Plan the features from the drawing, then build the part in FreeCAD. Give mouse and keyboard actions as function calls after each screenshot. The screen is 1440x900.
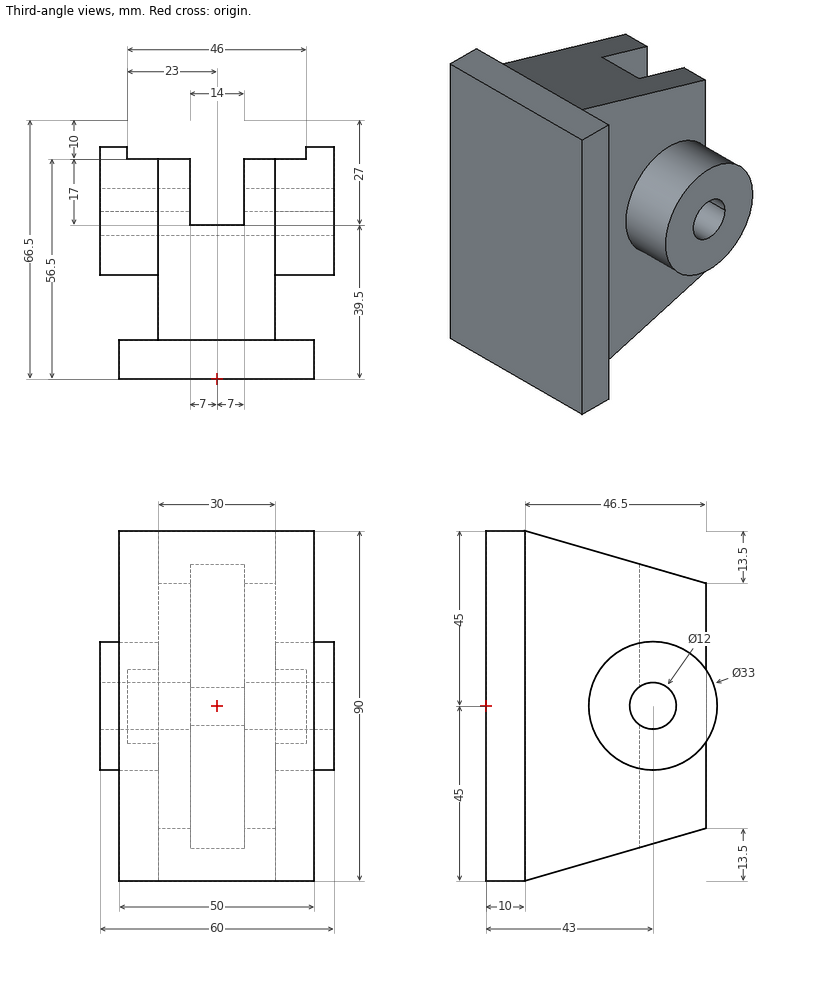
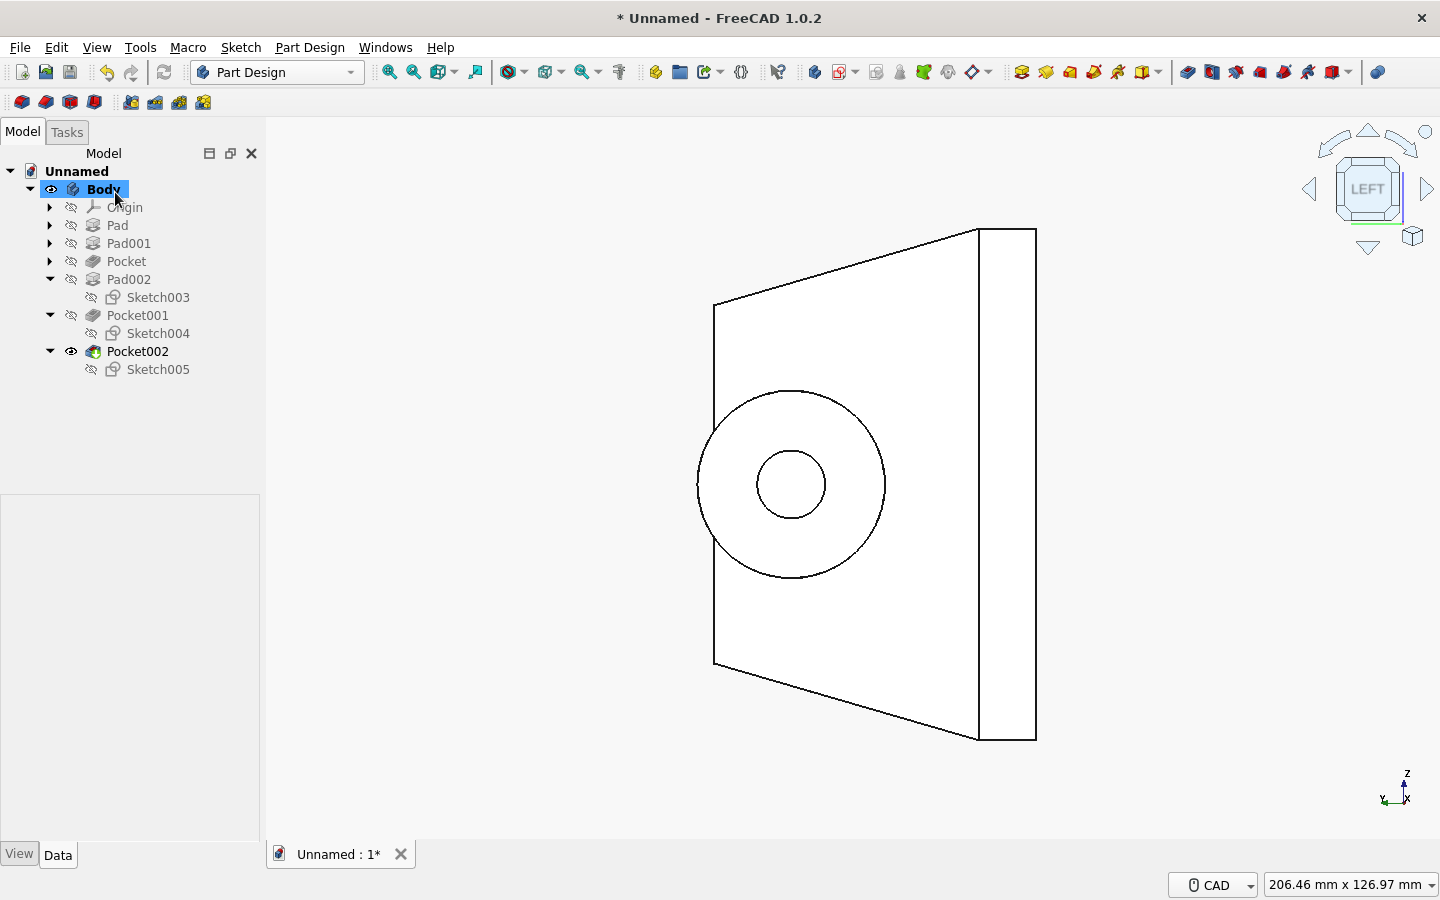
click(884, 630)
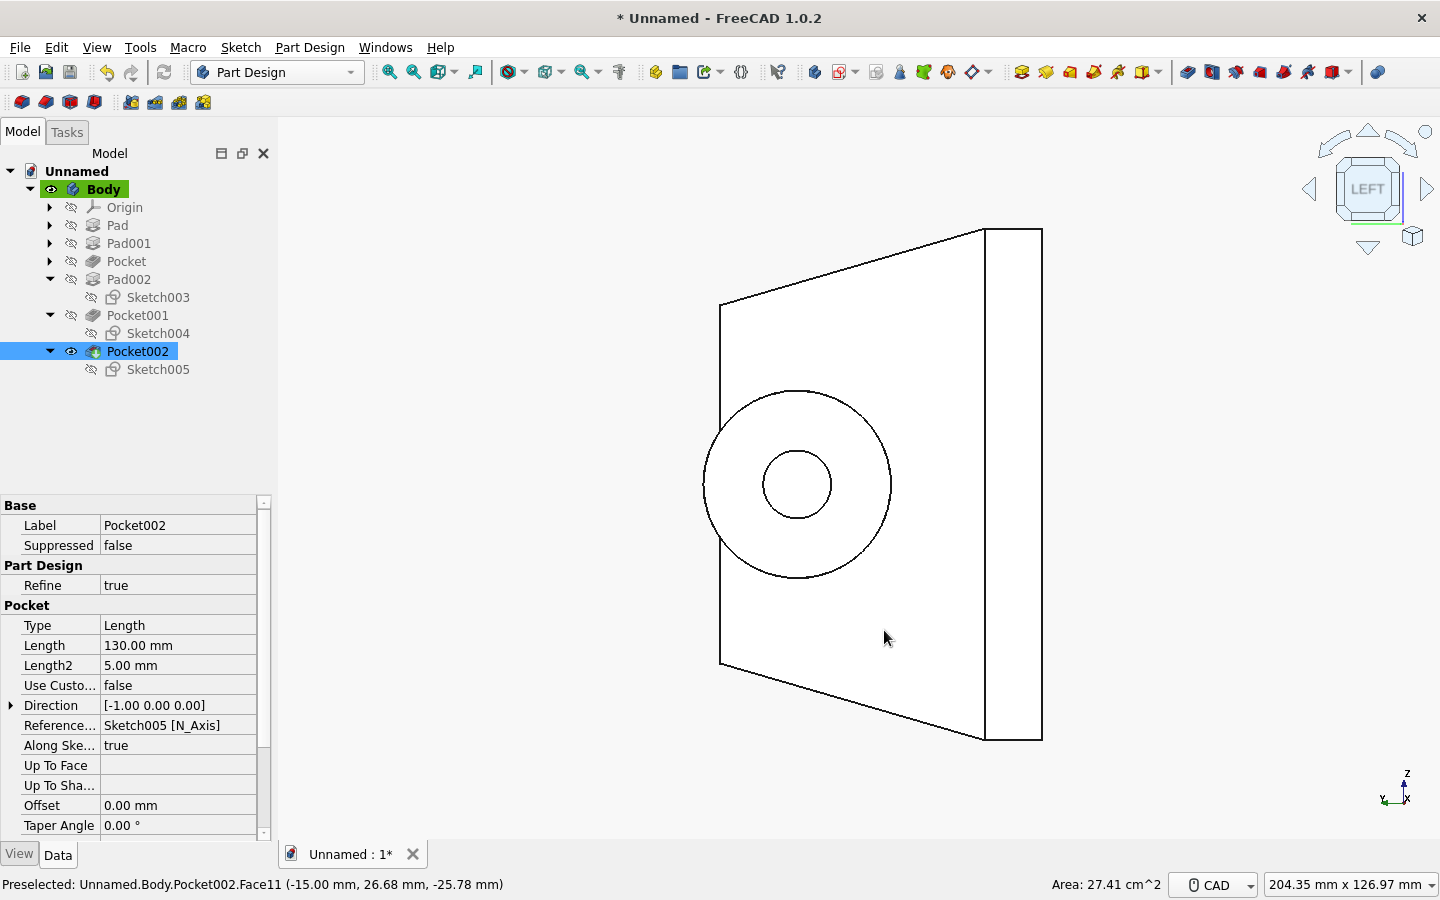
click(840, 72)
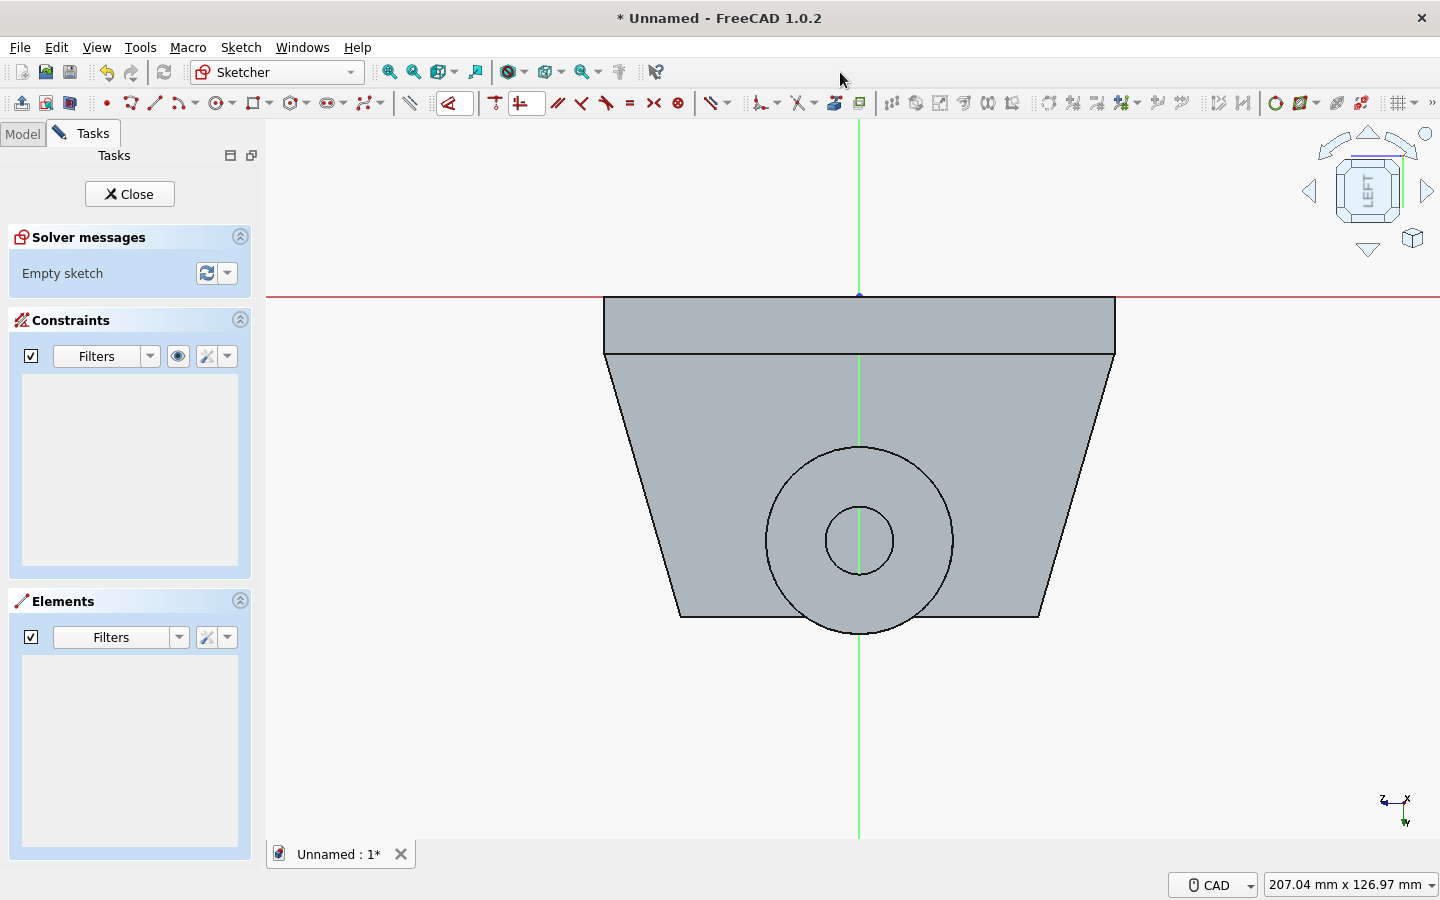
click(70, 104)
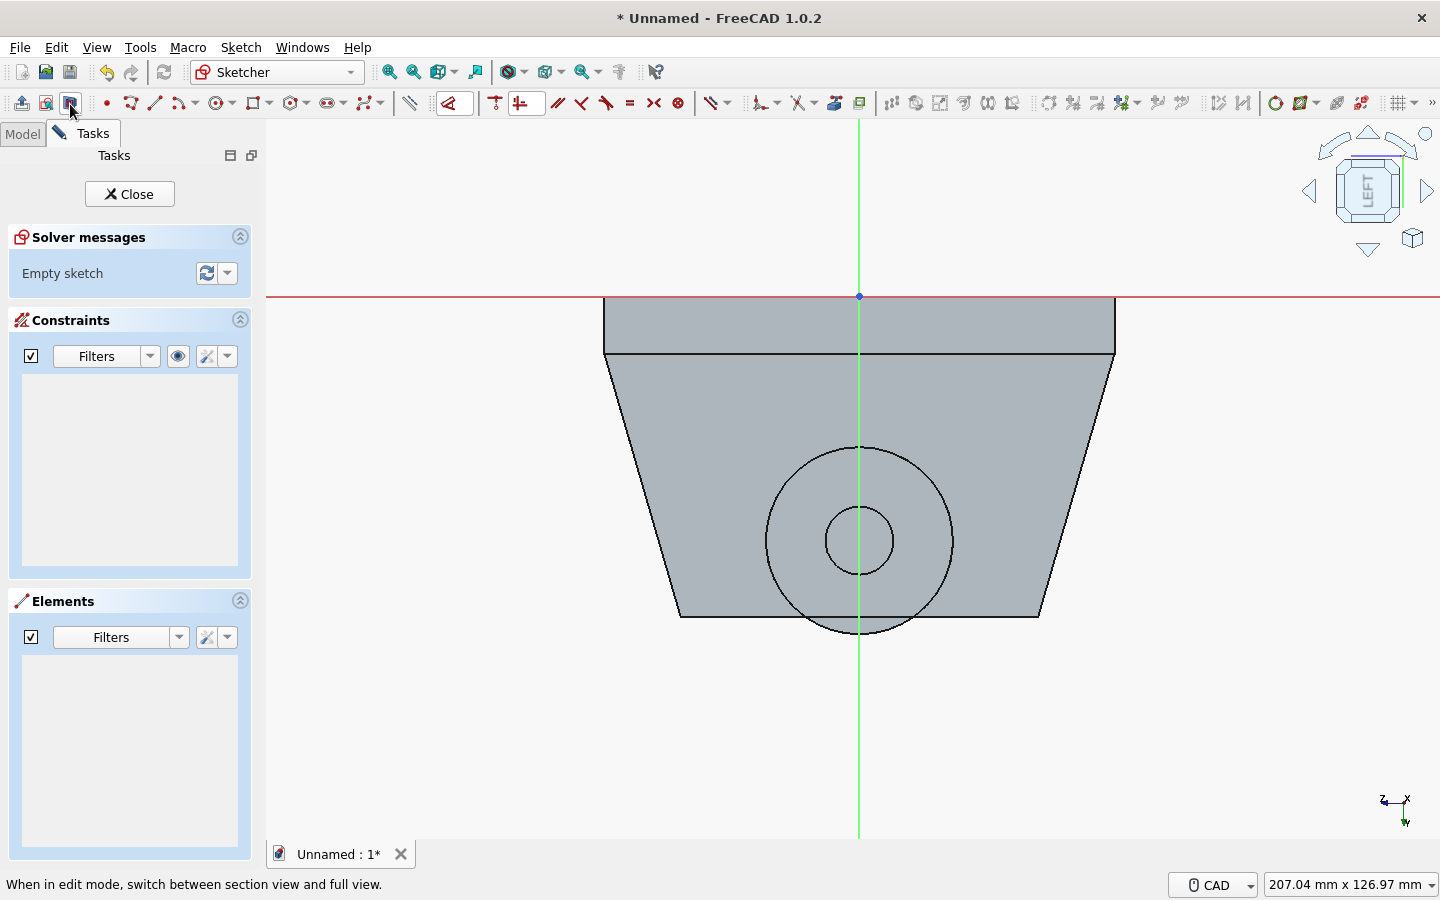
scroll(871, 550, up, 10)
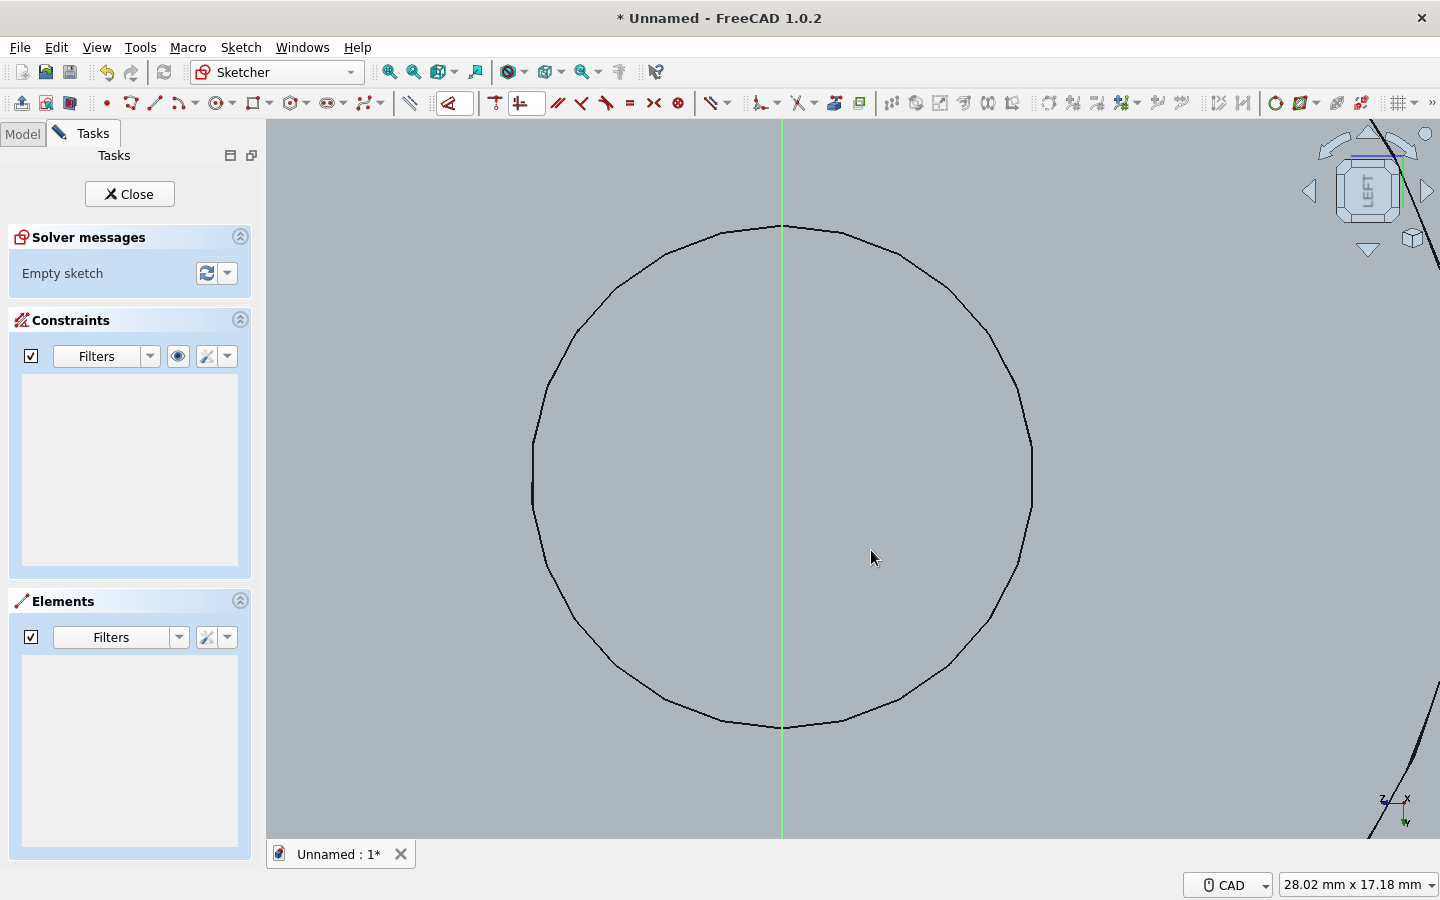
click(216, 104)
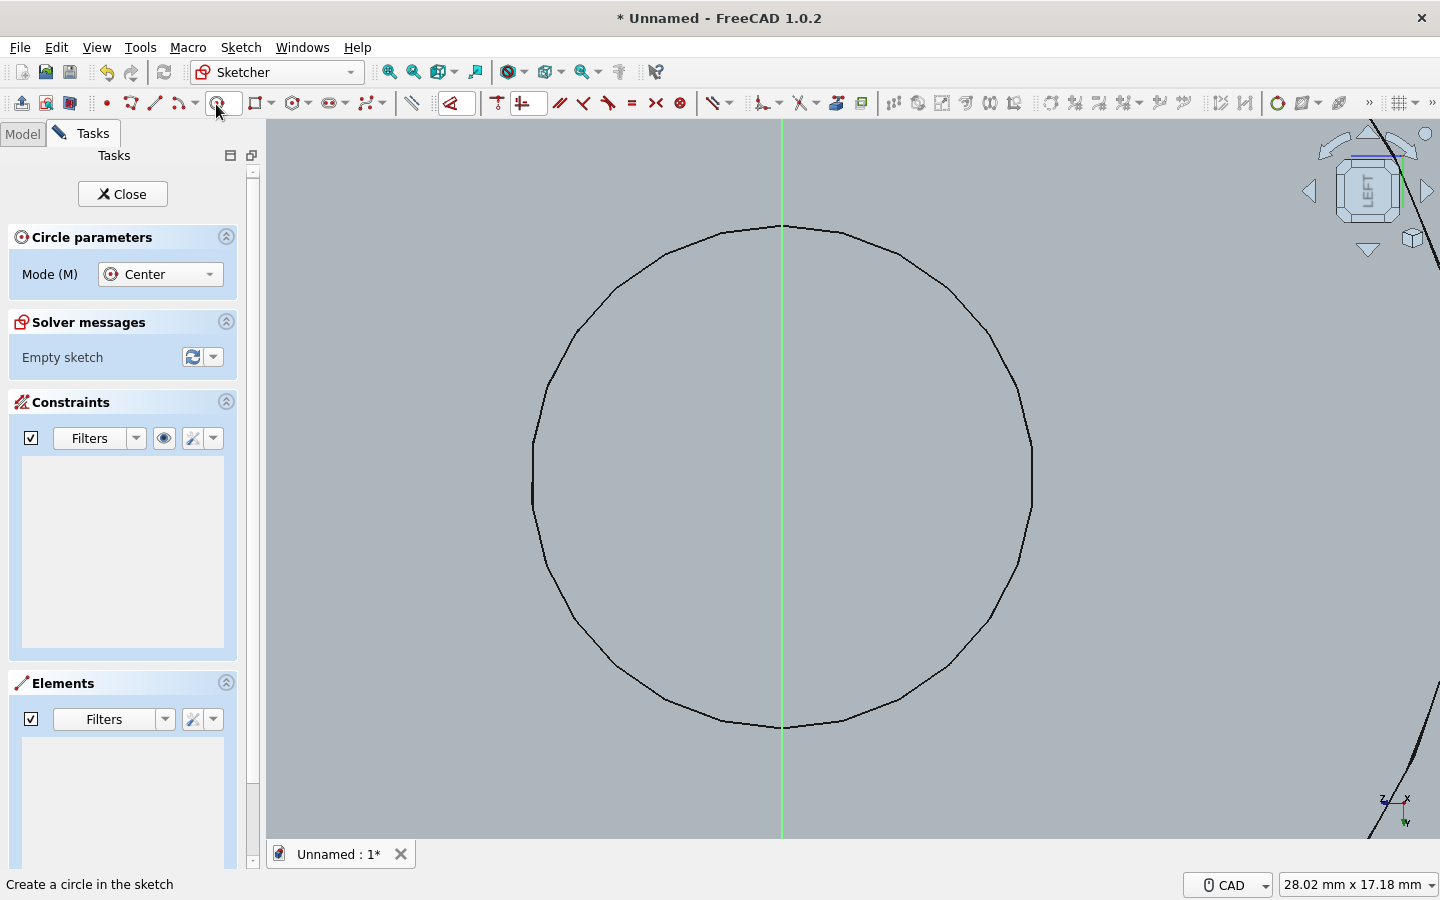
click(782, 477)
click(960, 299)
key(Escape)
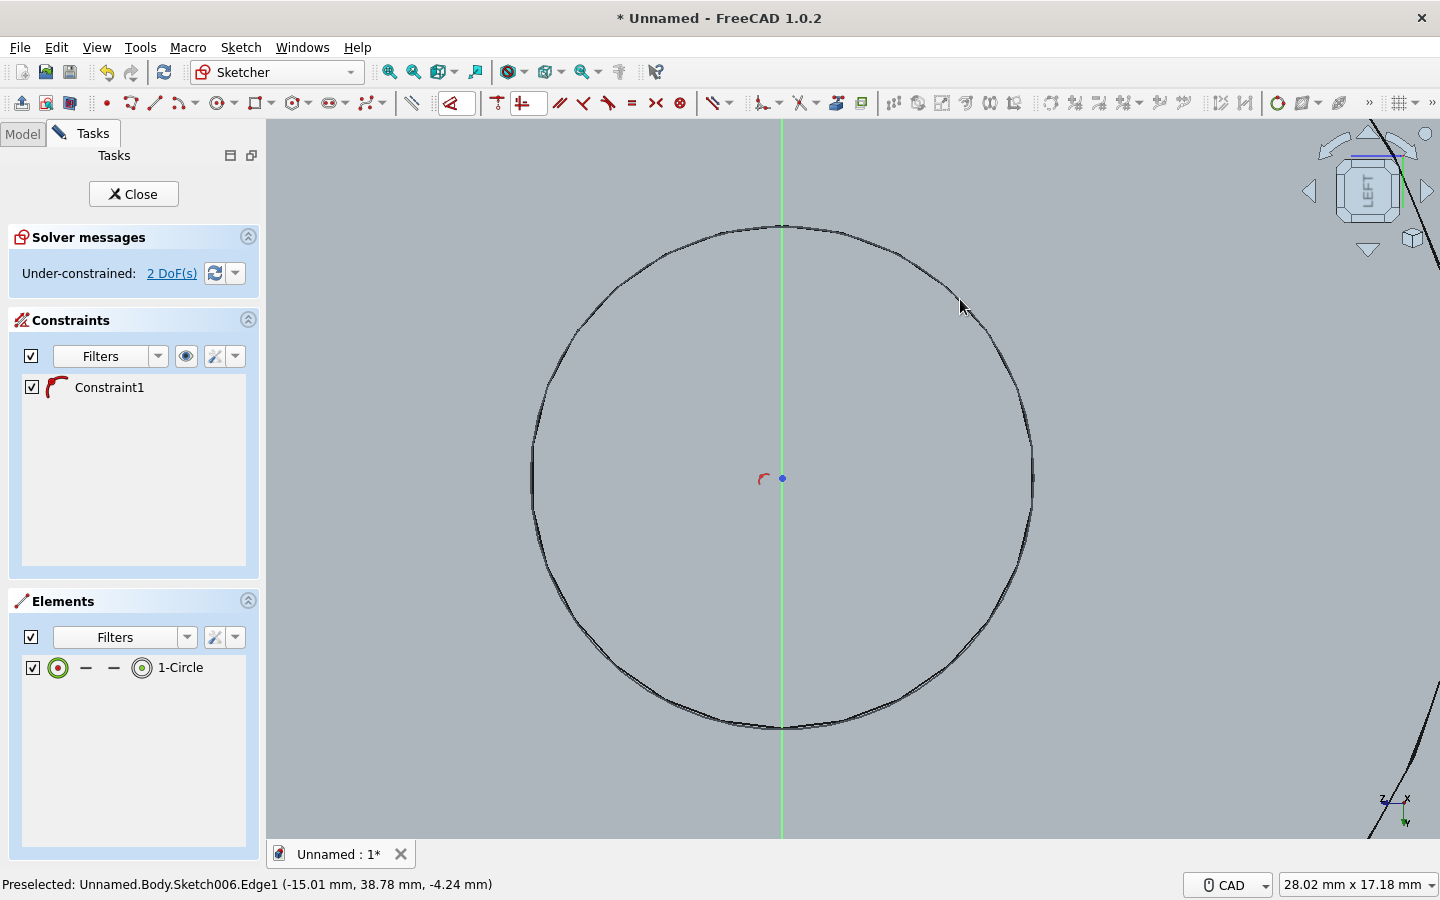
click(960, 300)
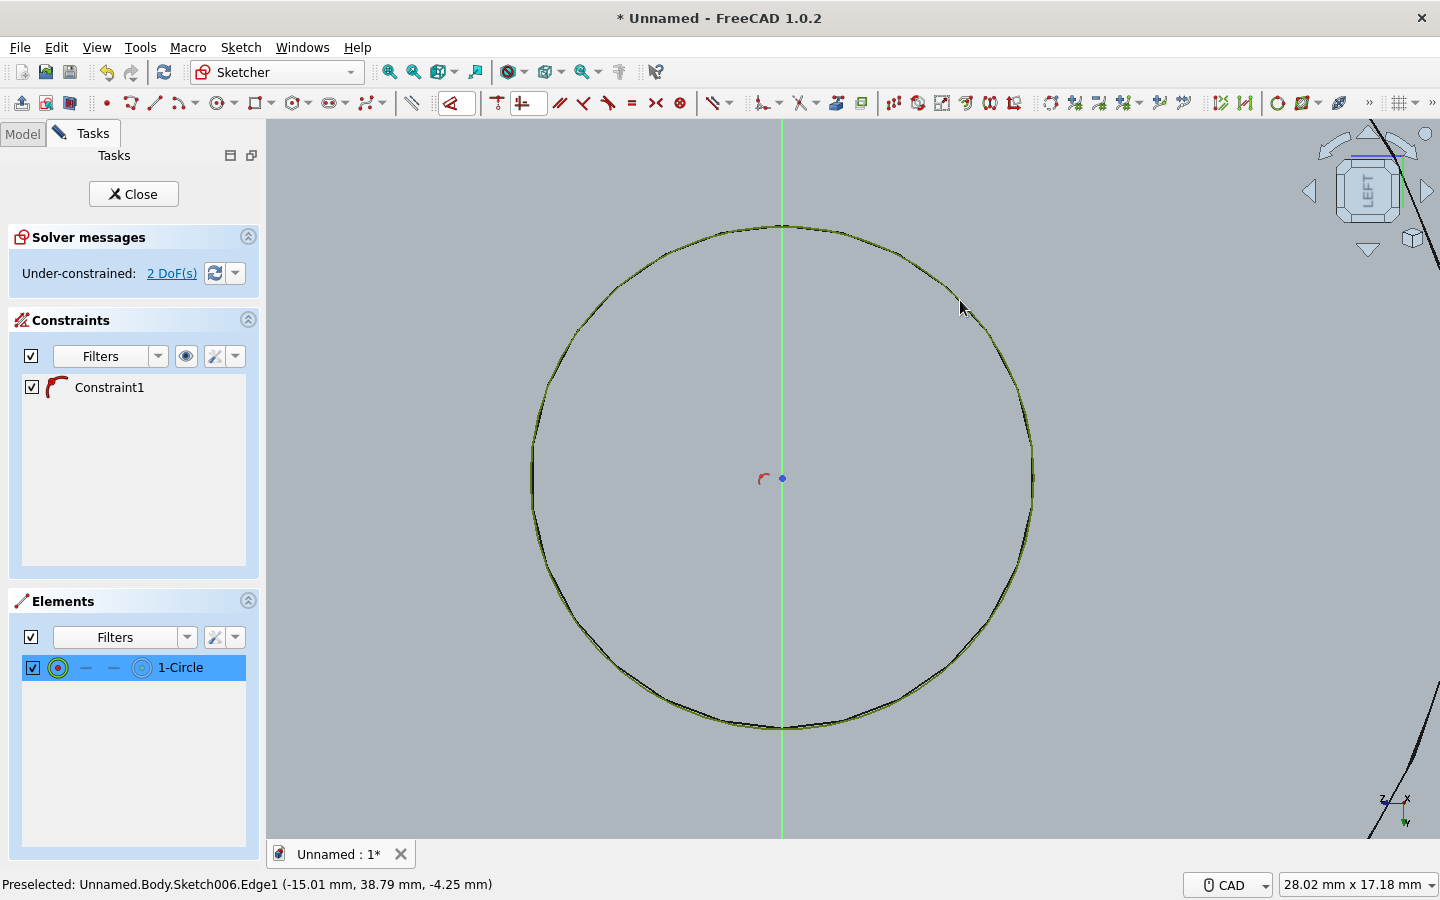
click(470, 104)